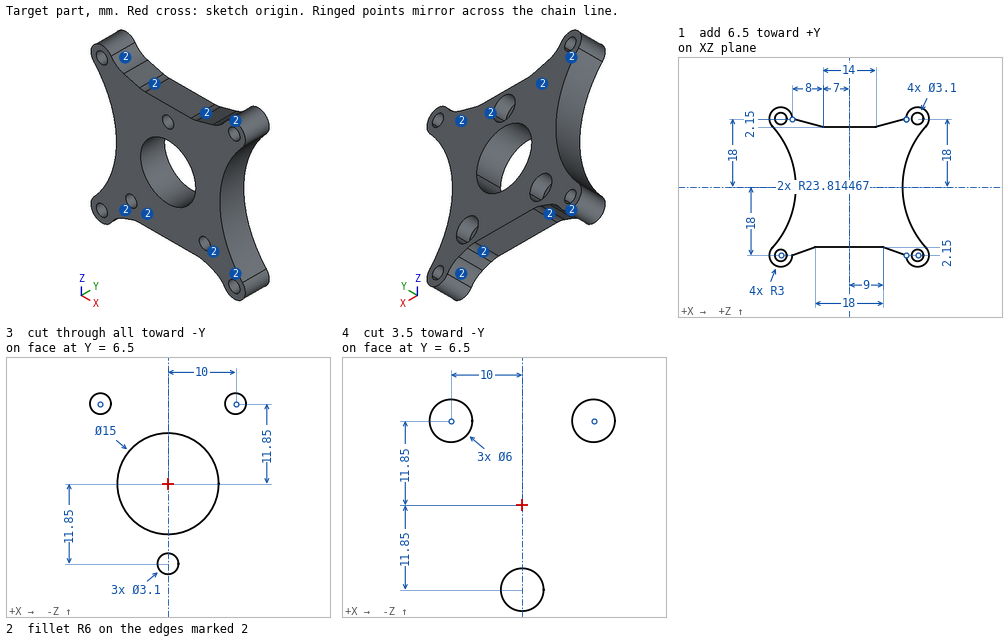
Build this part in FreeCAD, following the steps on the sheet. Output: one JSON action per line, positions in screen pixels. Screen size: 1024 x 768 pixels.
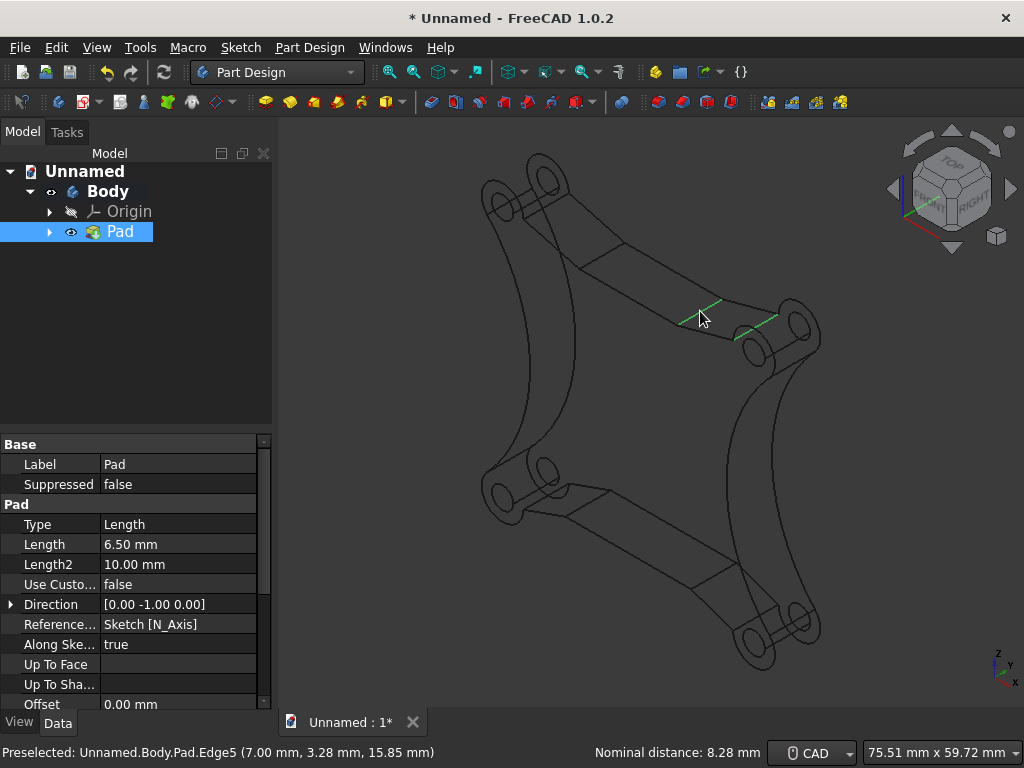
{"action": "left_click", "coordinate": [602, 255], "text": "ctrl"}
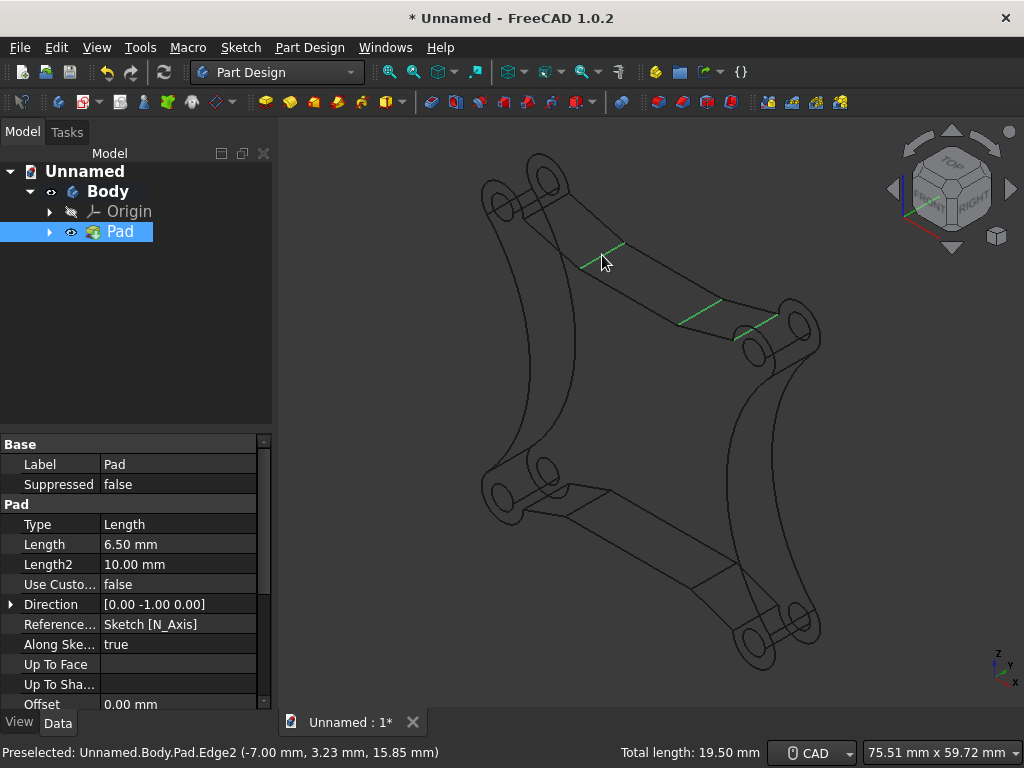
{"action": "left_click", "coordinate": [546, 205], "text": "ctrl"}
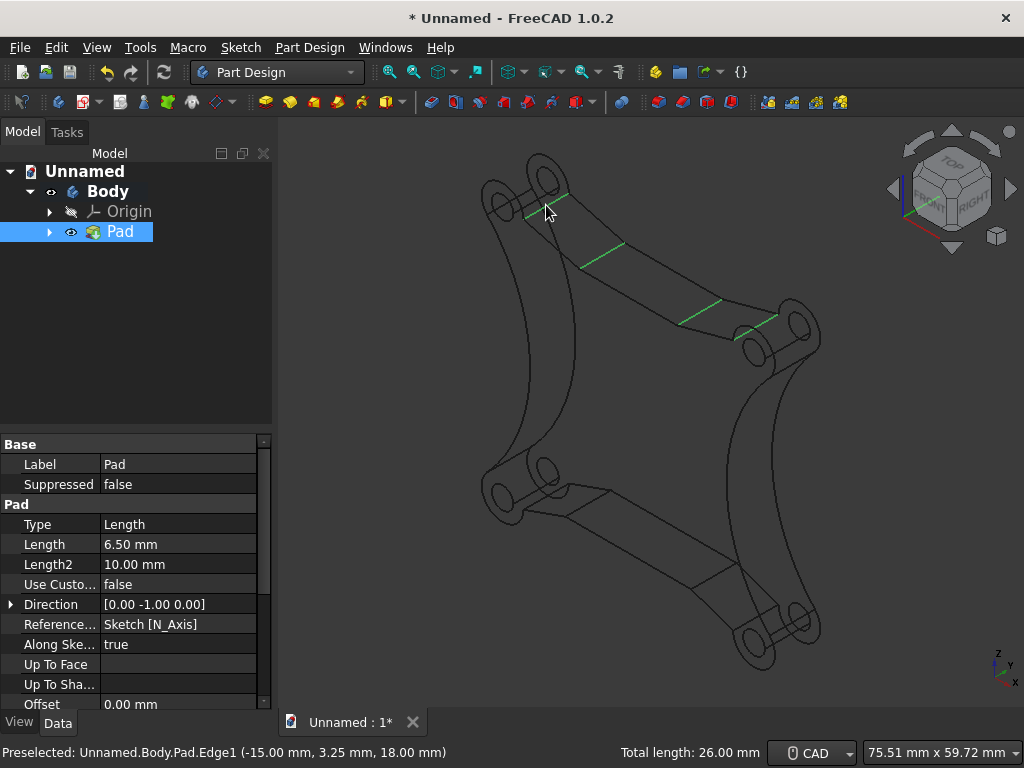
{"action": "left_click", "coordinate": [546, 496], "text": "ctrl"}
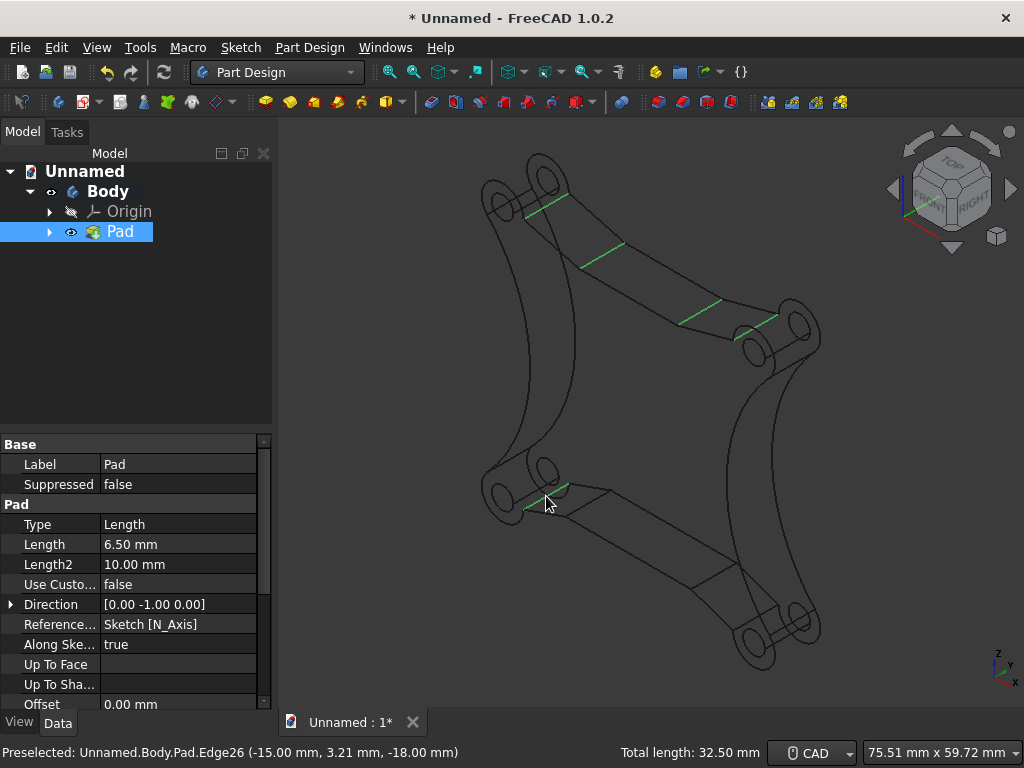
{"action": "left_click", "coordinate": [588, 503], "text": "ctrl"}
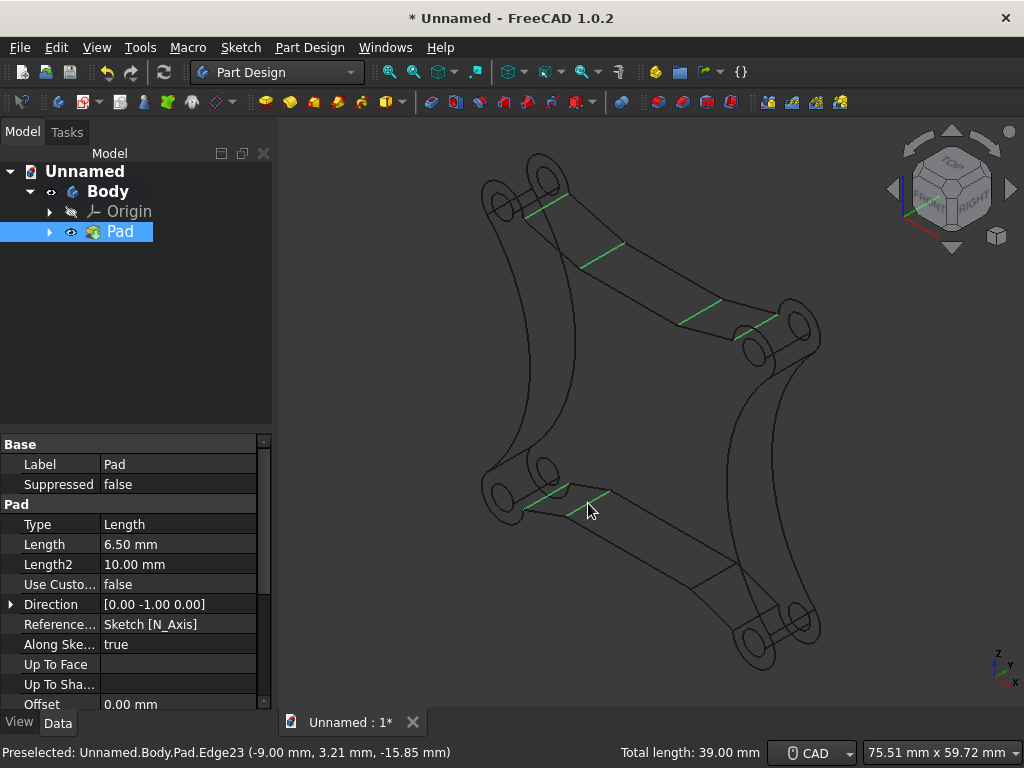
{"action": "left_click", "coordinate": [714, 575], "text": "ctrl"}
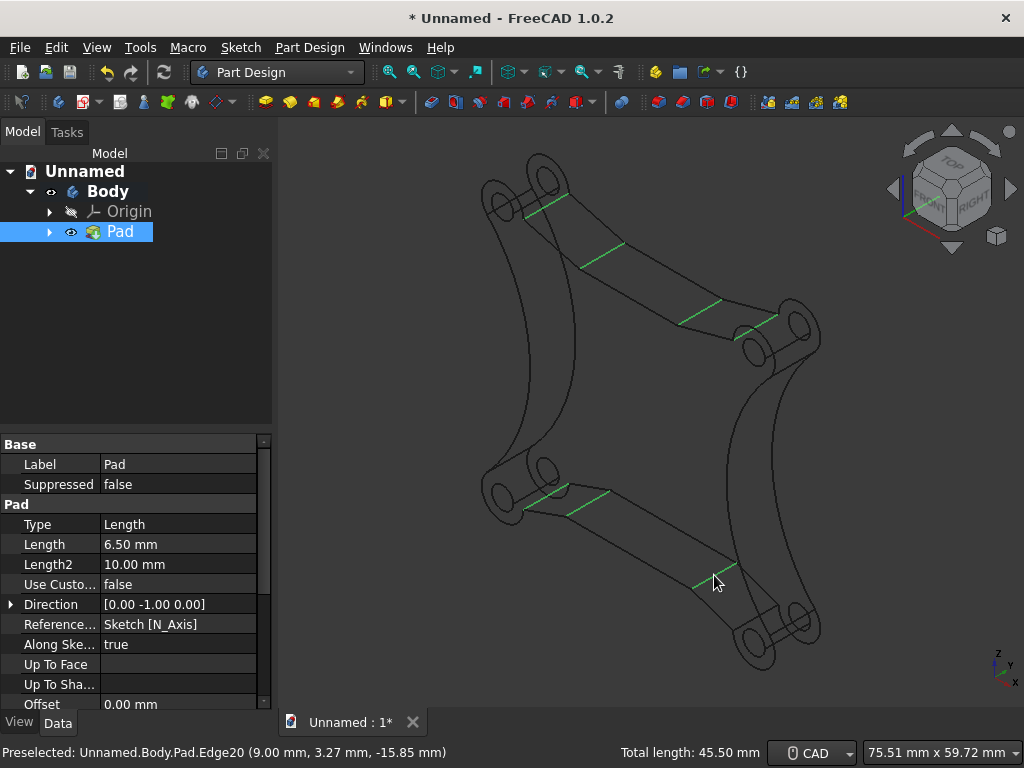
{"action": "left_click", "coordinate": [751, 619], "text": "ctrl"}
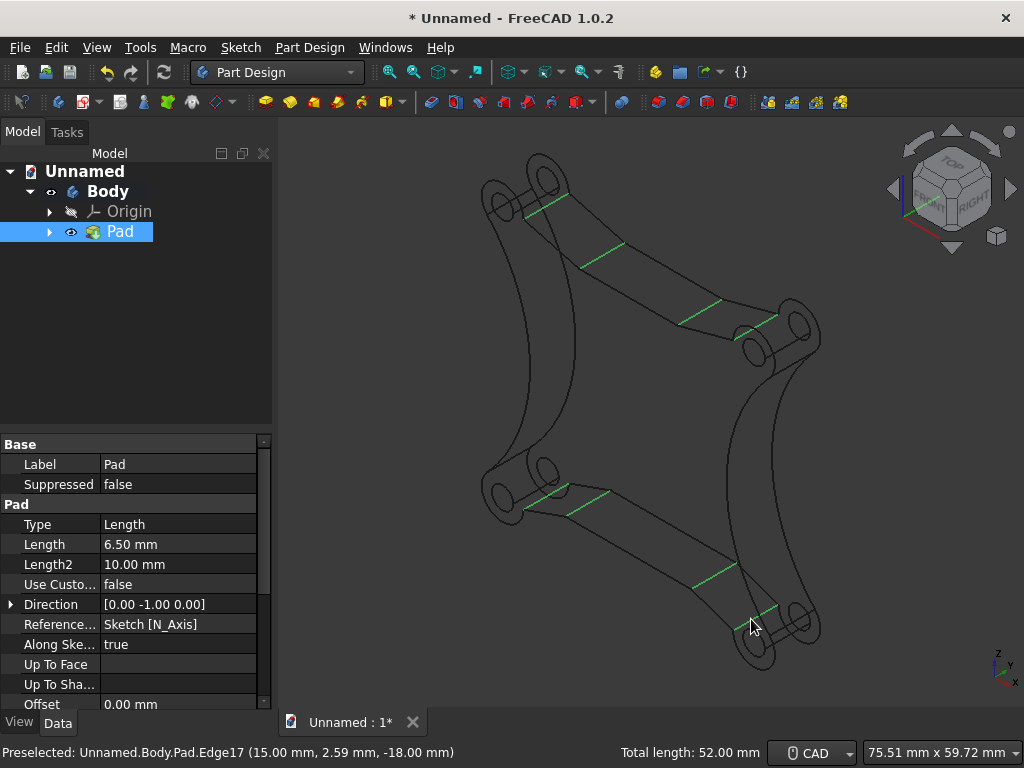
{"action": "key", "text": "v 1"}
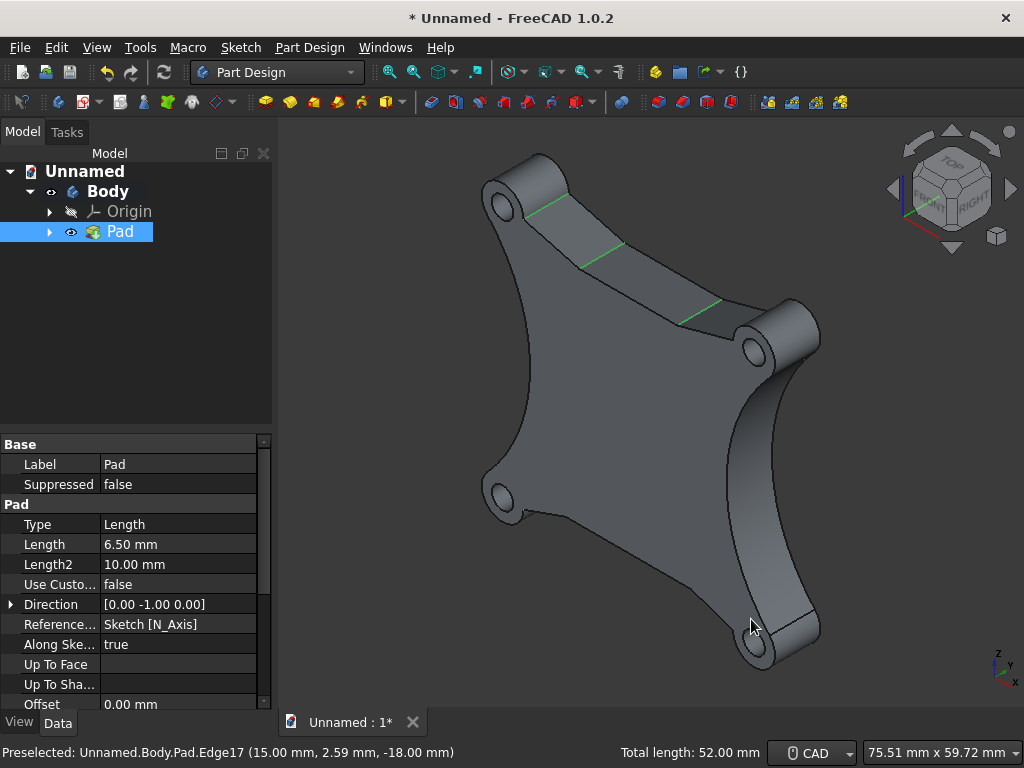
{"action": "left_click", "coordinate": [660, 102]}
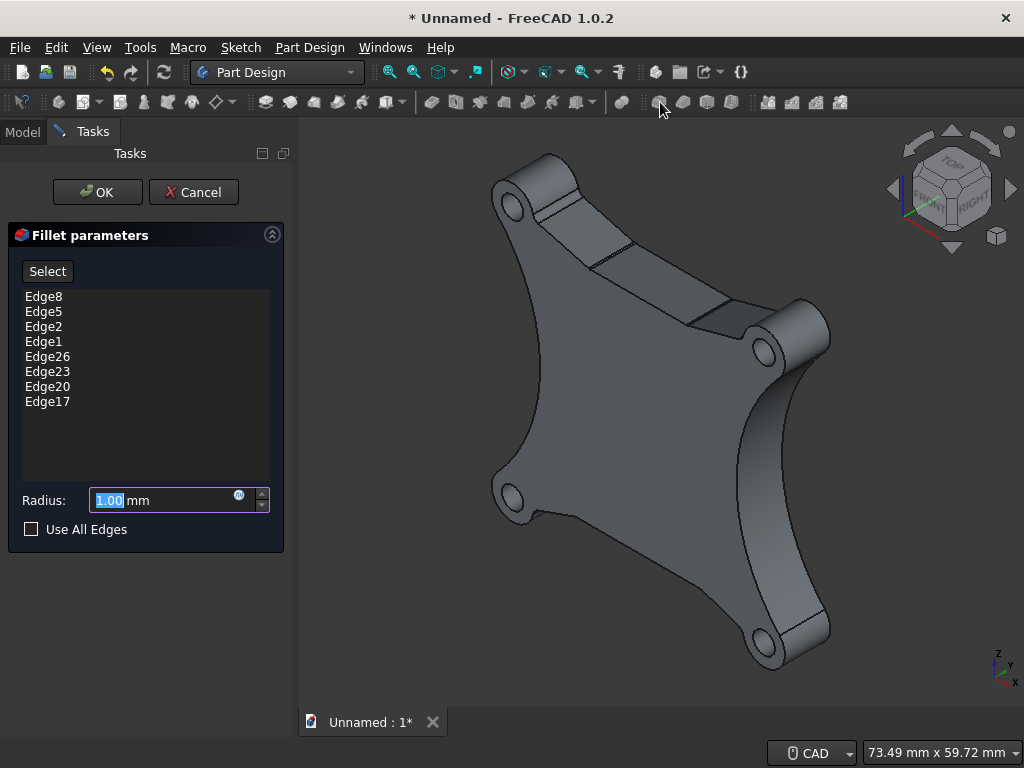
{"action": "type", "text": "6"}
{"action": "key", "text": "Tab"}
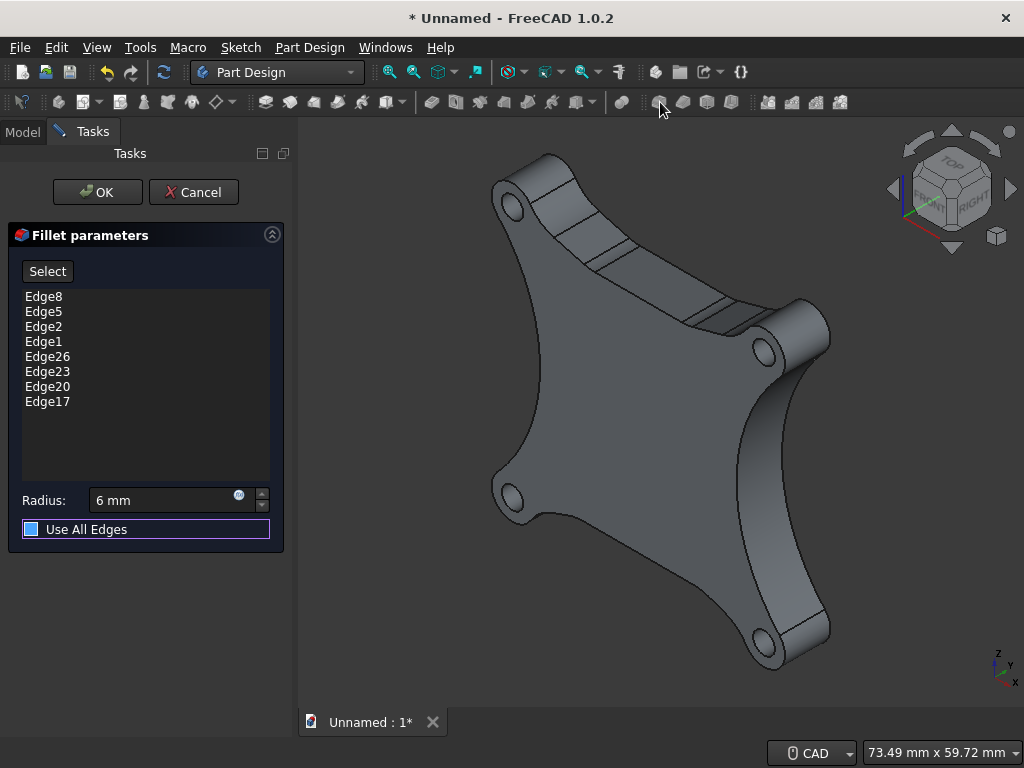
{"action": "left_click", "coordinate": [98, 192]}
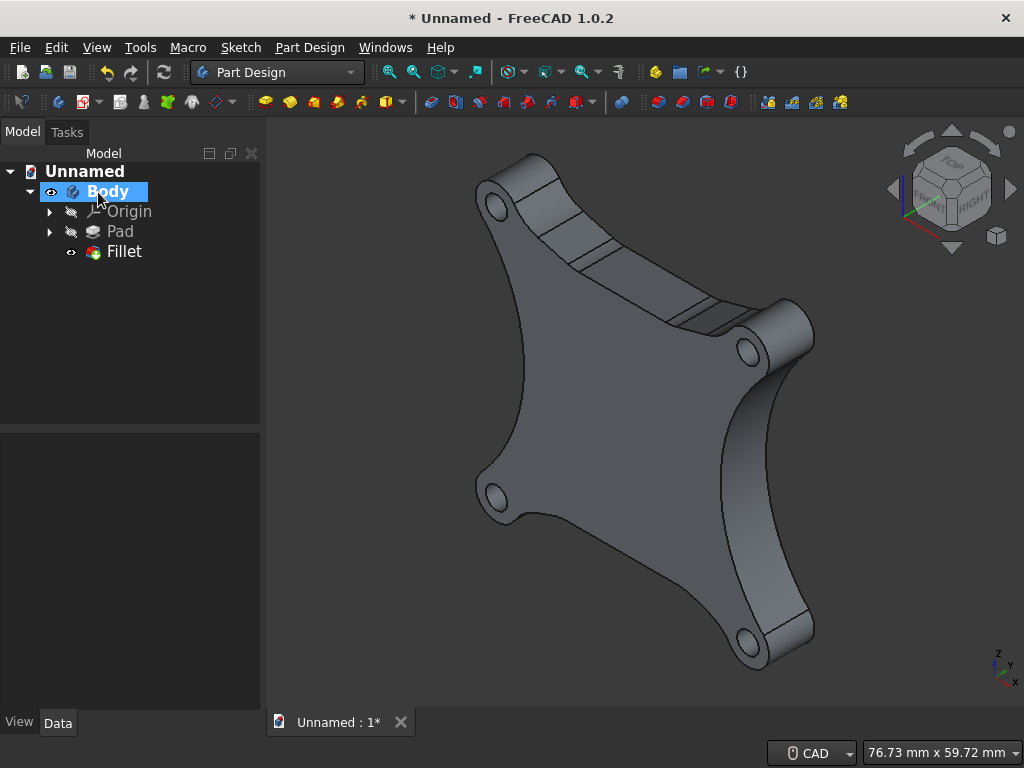
{"action": "key", "text": "4"}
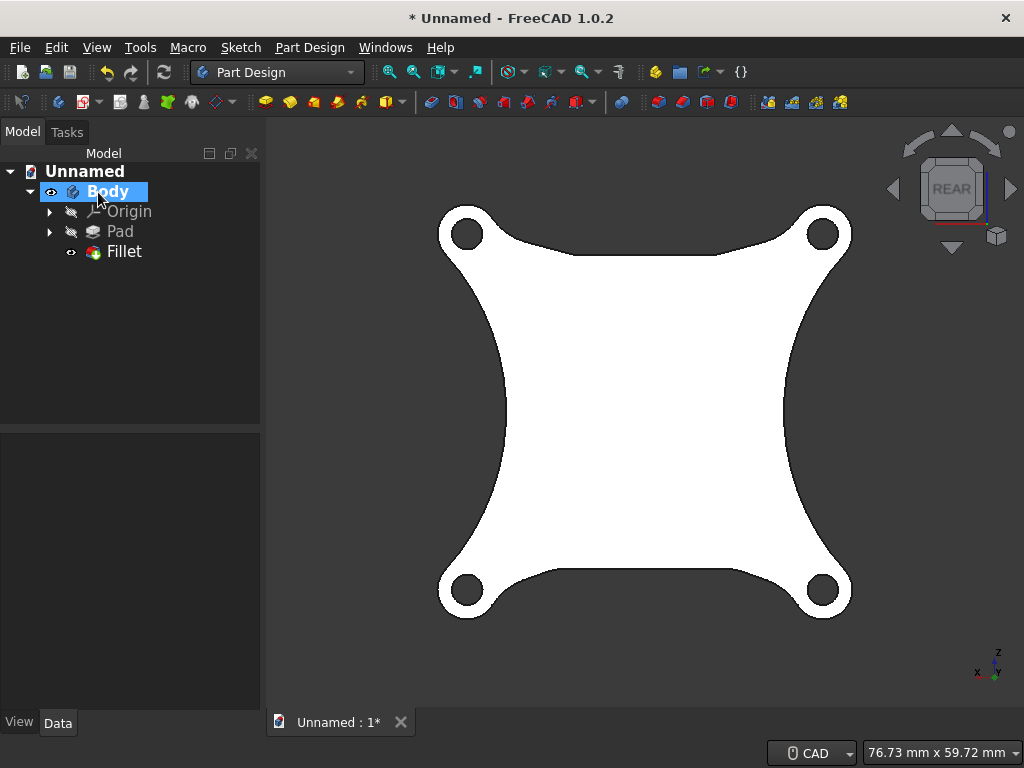
{"action": "left_click", "coordinate": [645, 411]}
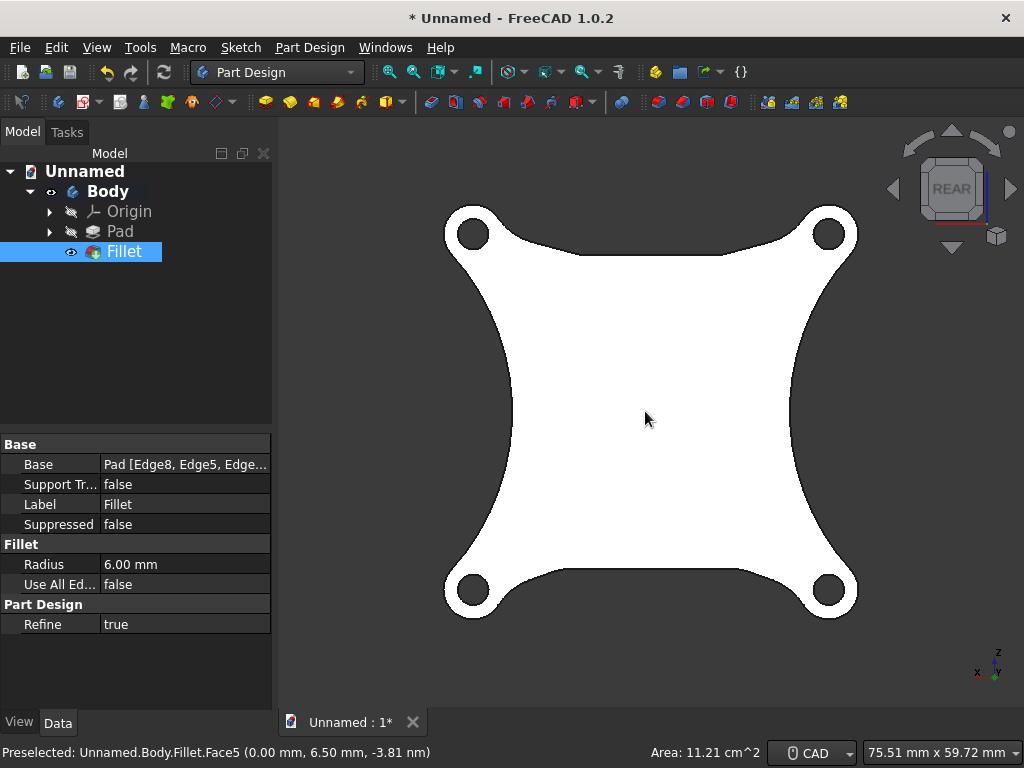
{"action": "left_click", "coordinate": [84, 102]}